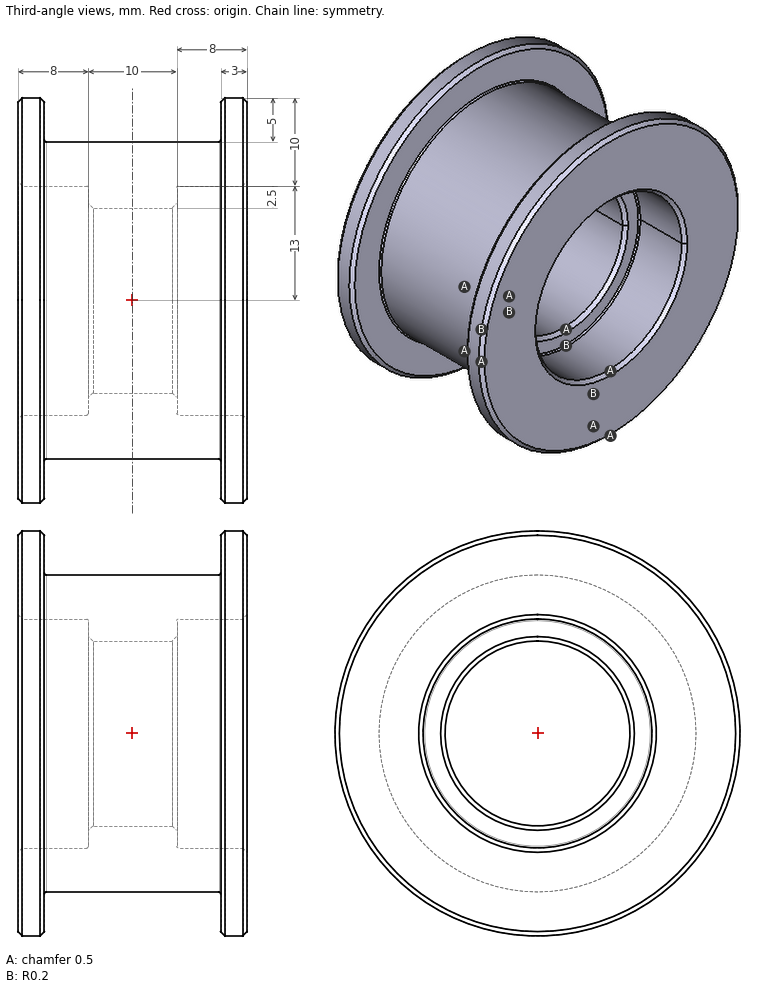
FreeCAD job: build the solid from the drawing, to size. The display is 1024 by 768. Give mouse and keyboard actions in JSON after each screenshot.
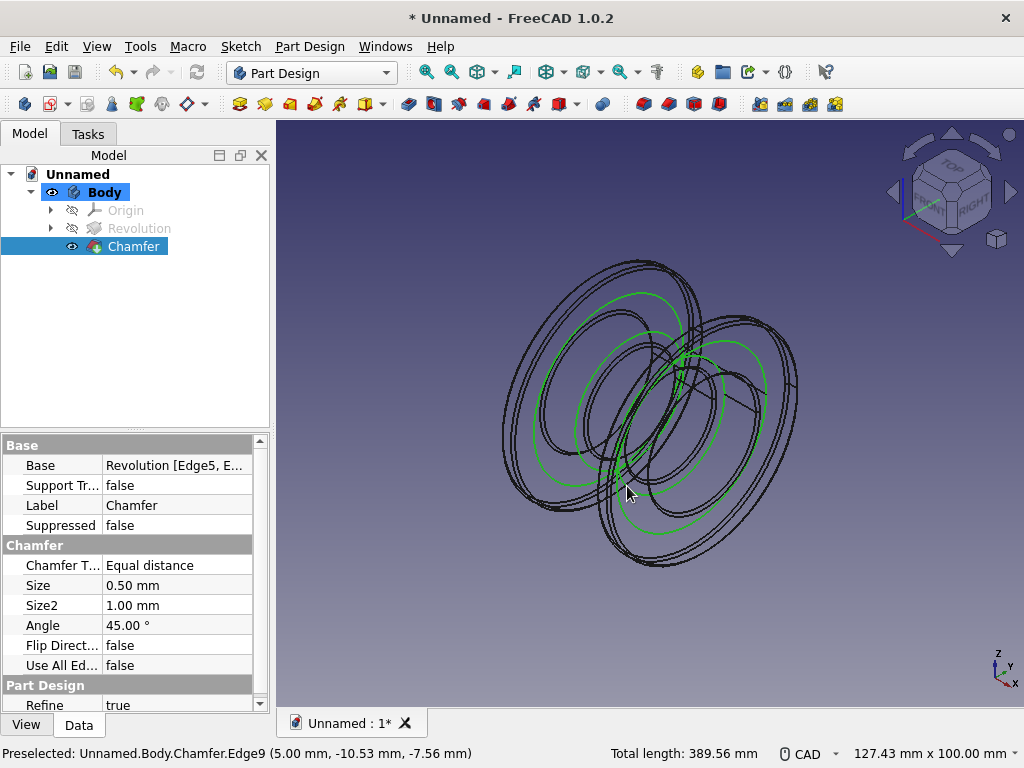
{"action": "key", "text": "v 1"}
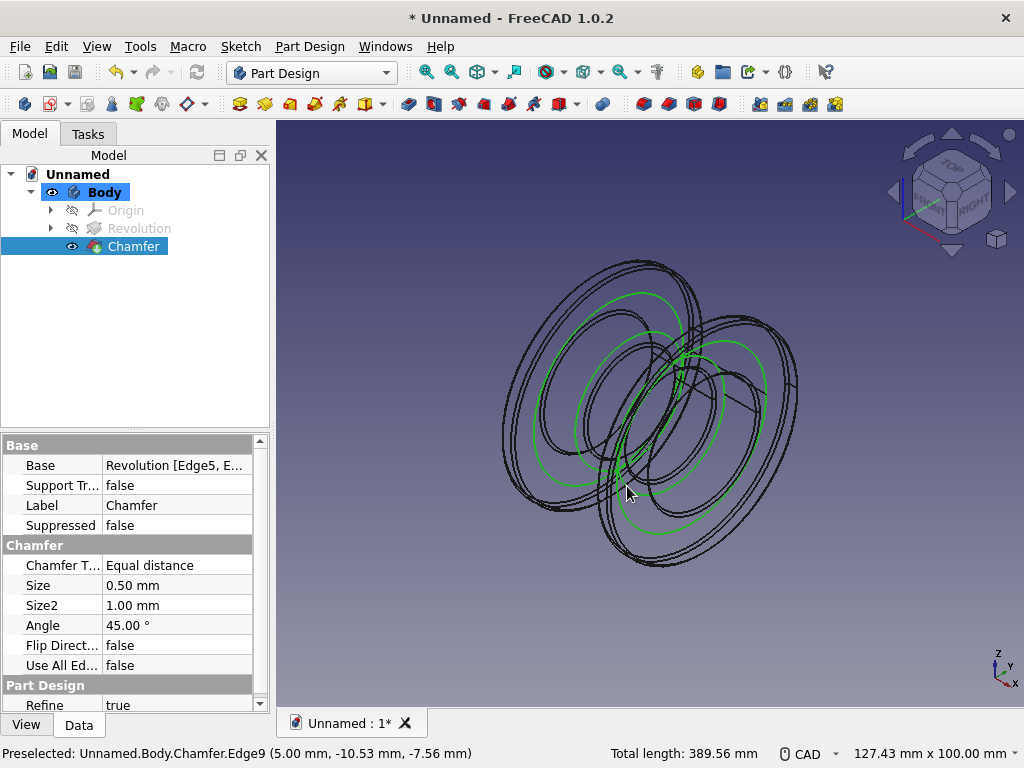
{"action": "left_click", "coordinate": [644, 104]}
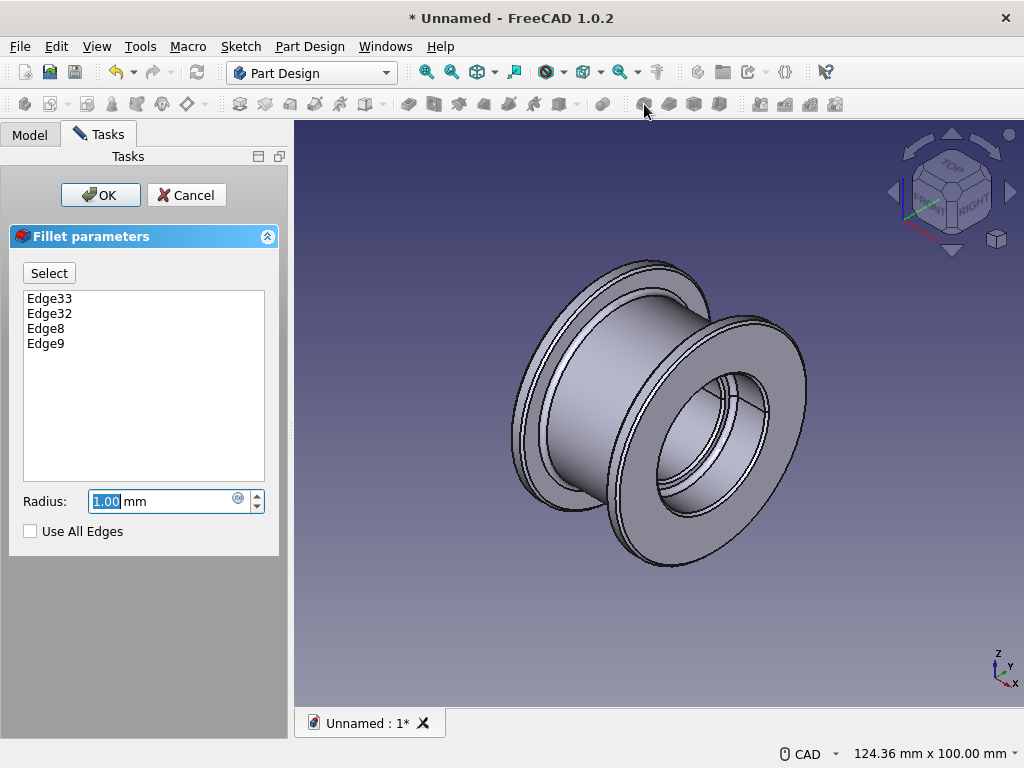
{"action": "type", "text": "0.2"}
{"action": "key", "text": "Tab"}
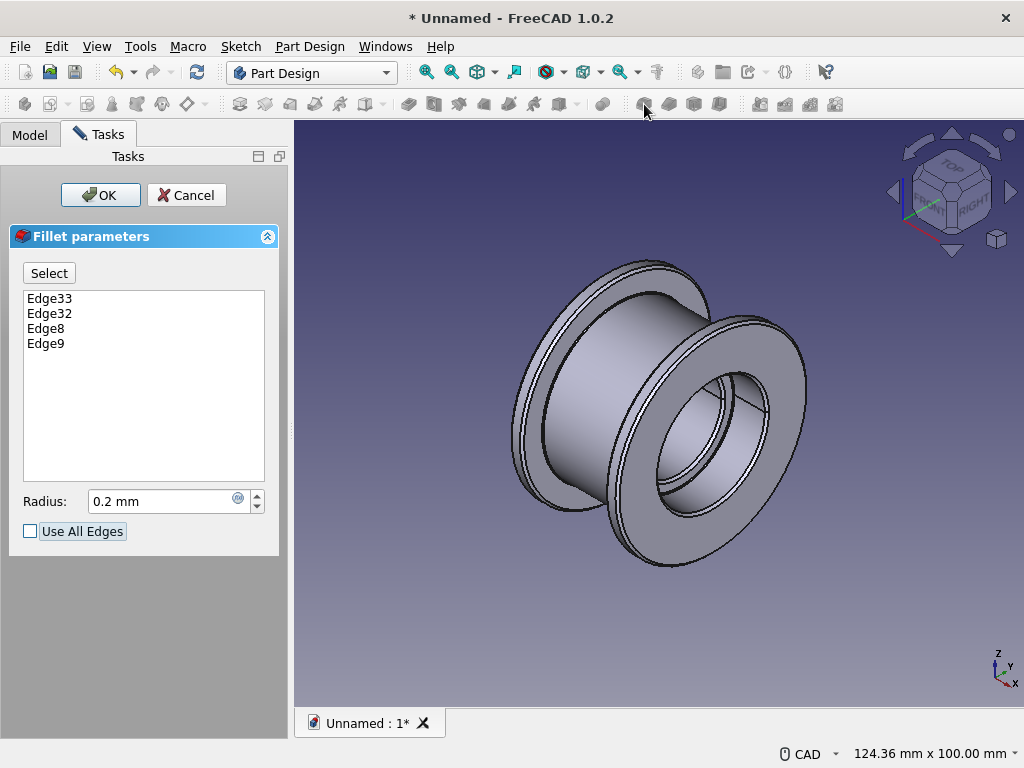
{"action": "left_click", "coordinate": [101, 195]}